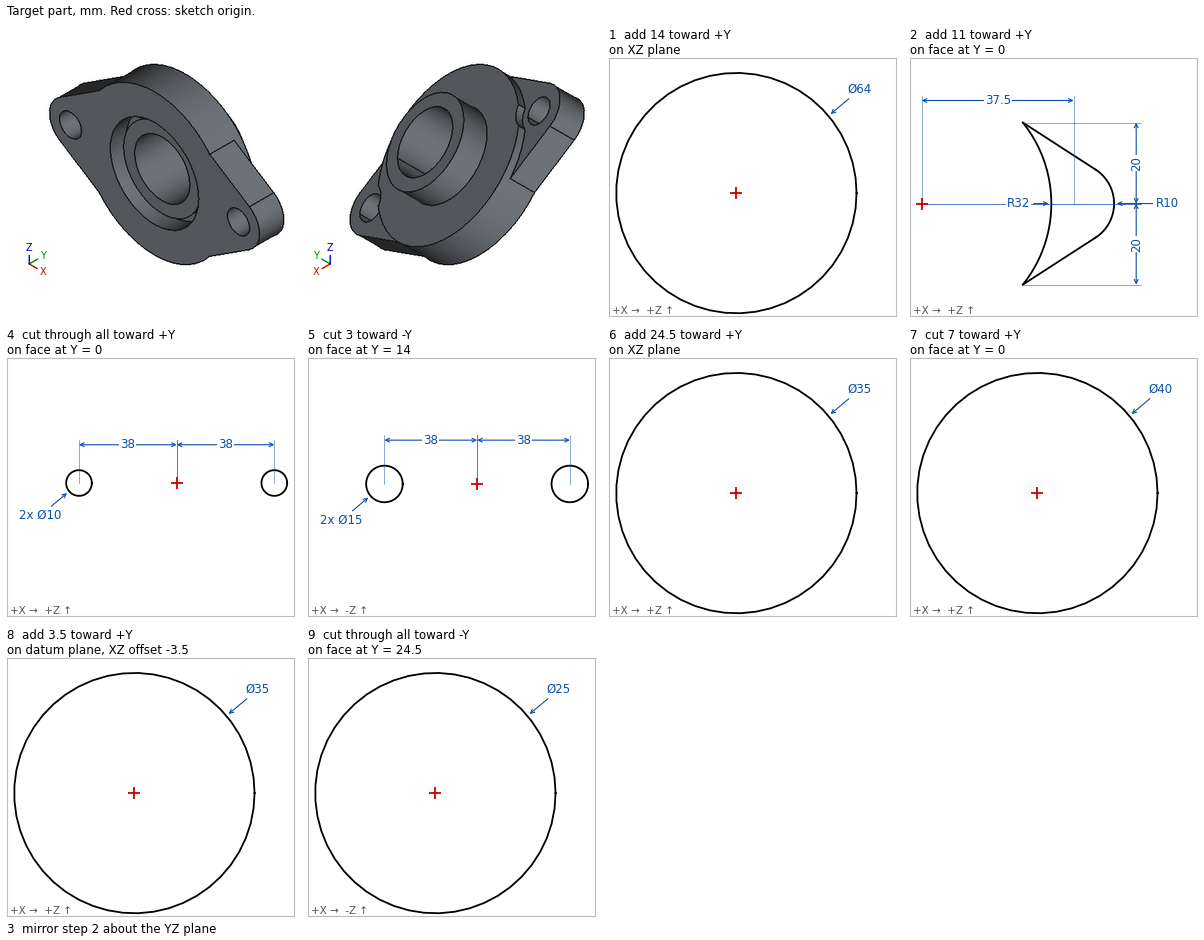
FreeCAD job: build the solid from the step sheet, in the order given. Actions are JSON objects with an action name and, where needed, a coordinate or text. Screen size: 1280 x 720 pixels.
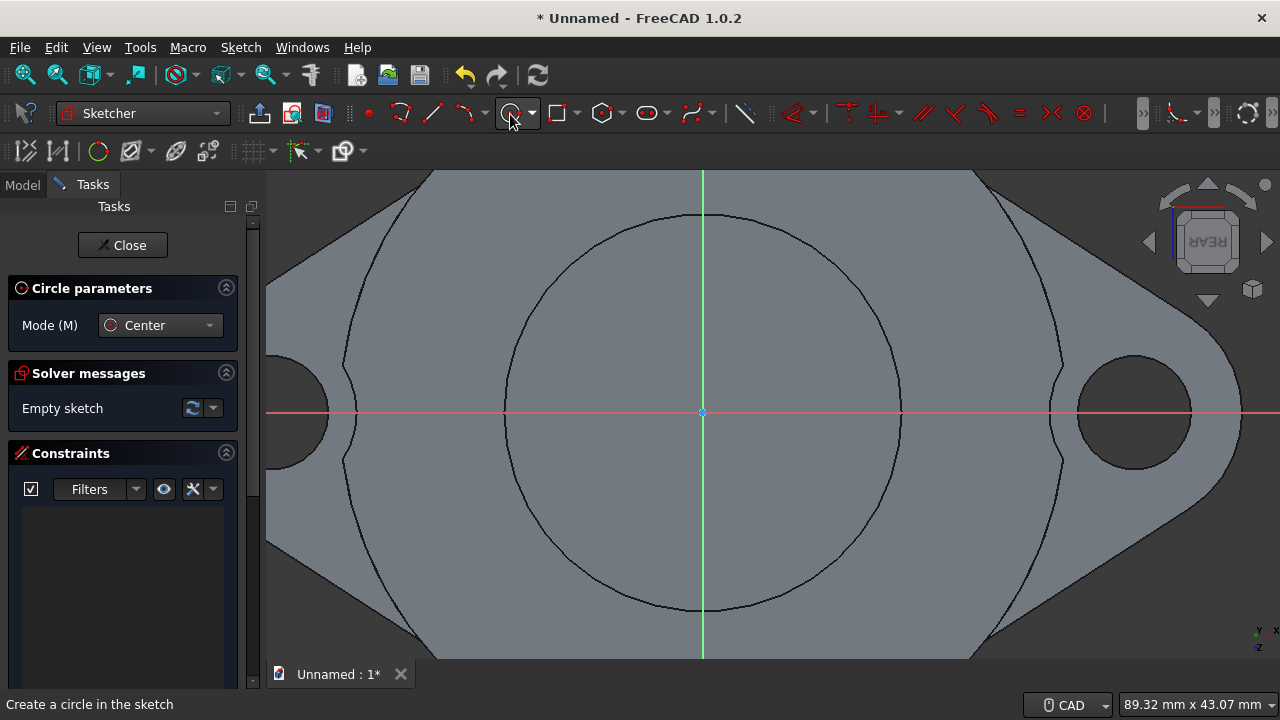
{"action": "left_click", "coordinate": [703, 413]}
{"action": "left_click", "coordinate": [803, 312]}
{"action": "key", "text": "Escape"}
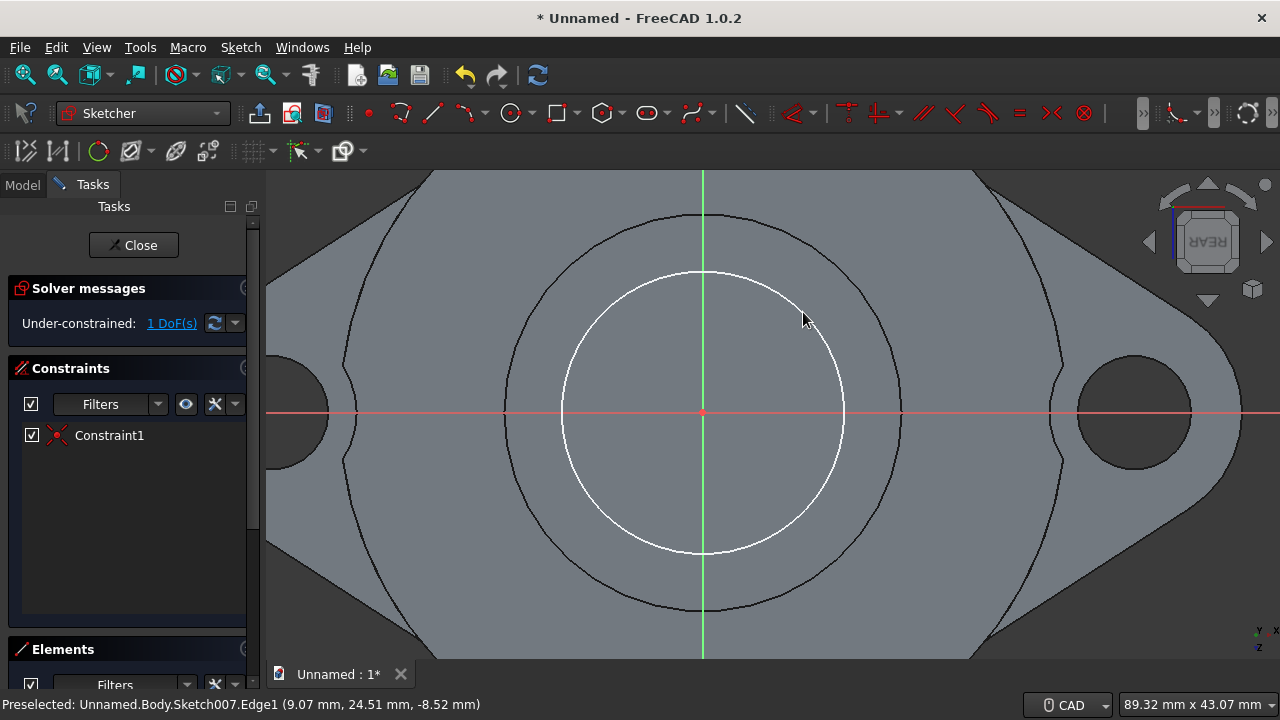
{"action": "left_click", "coordinate": [792, 114]}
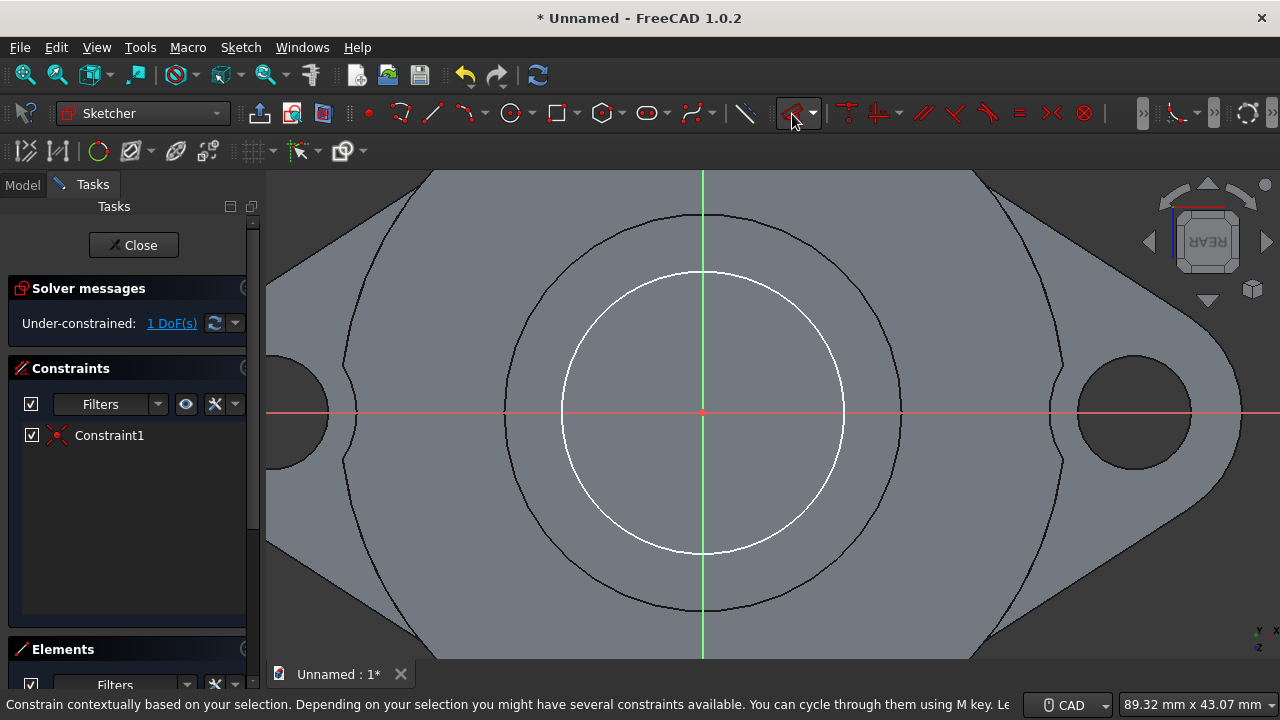
{"action": "left_click", "coordinate": [803, 313]}
{"action": "left_click", "coordinate": [826, 290]}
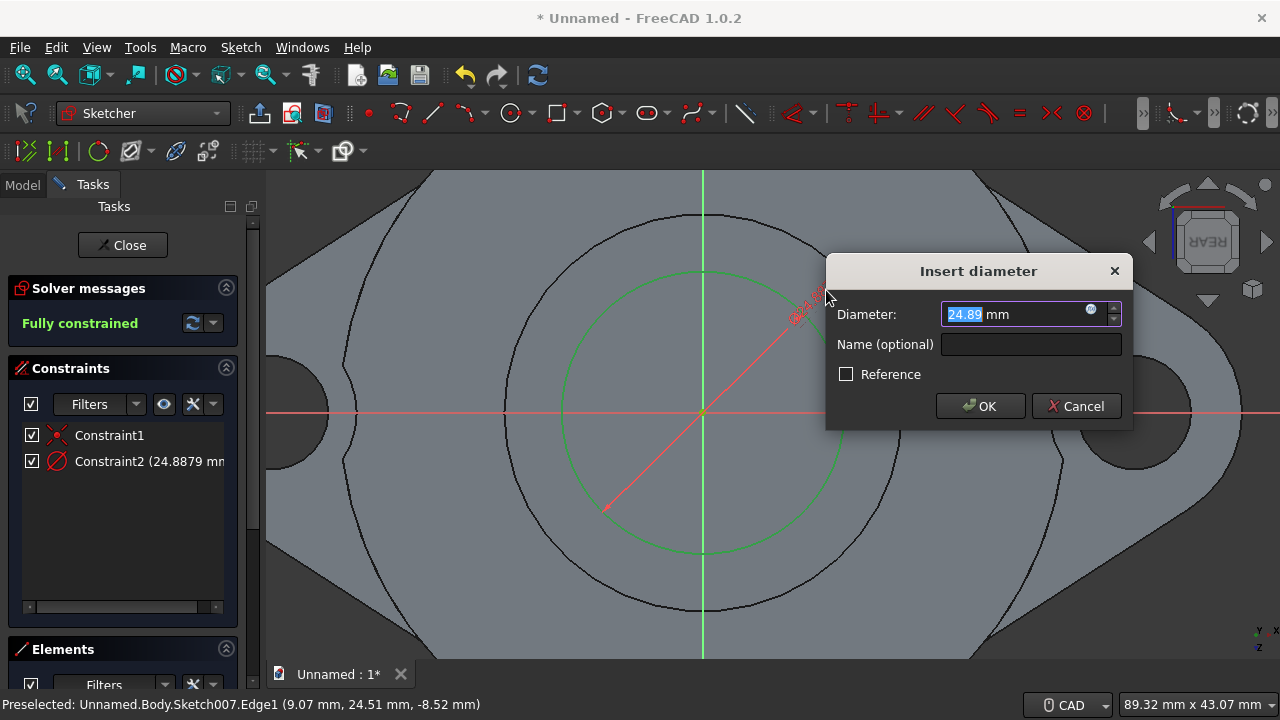
{"action": "type", "text": "25"}
{"action": "key", "text": "Return"}
{"action": "key", "text": "Escape"}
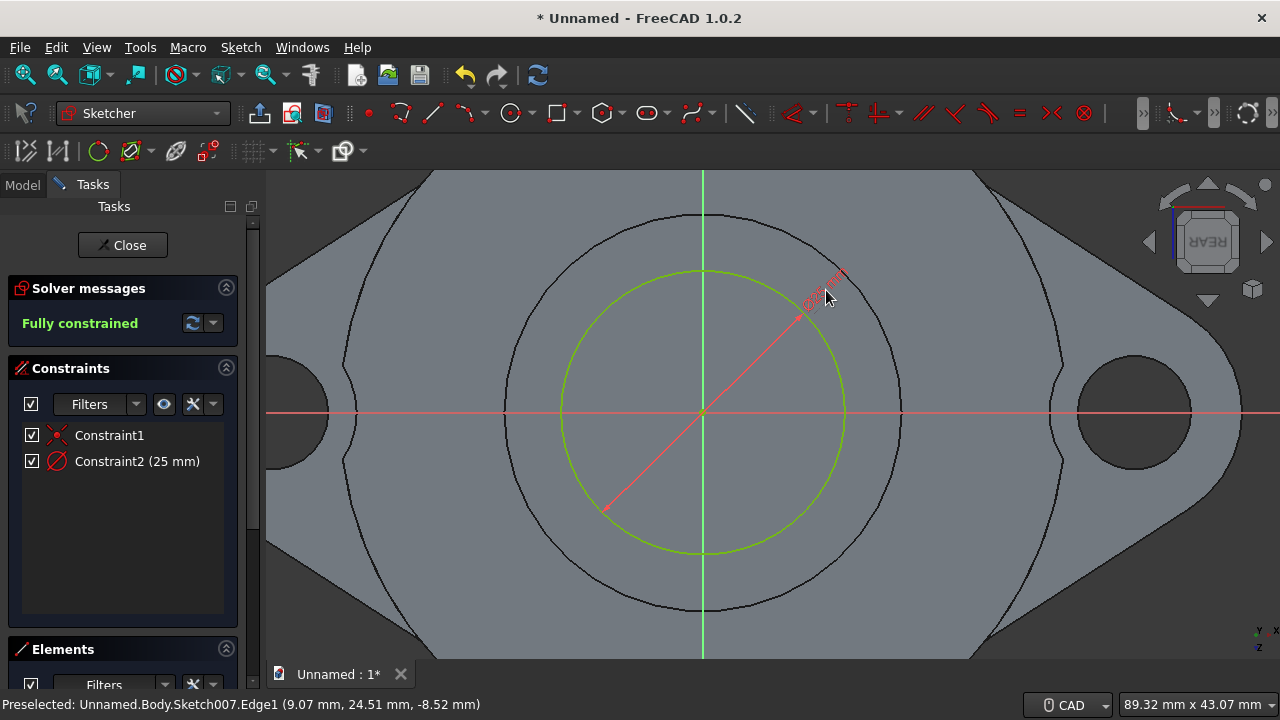
{"action": "left_click", "coordinate": [123, 245]}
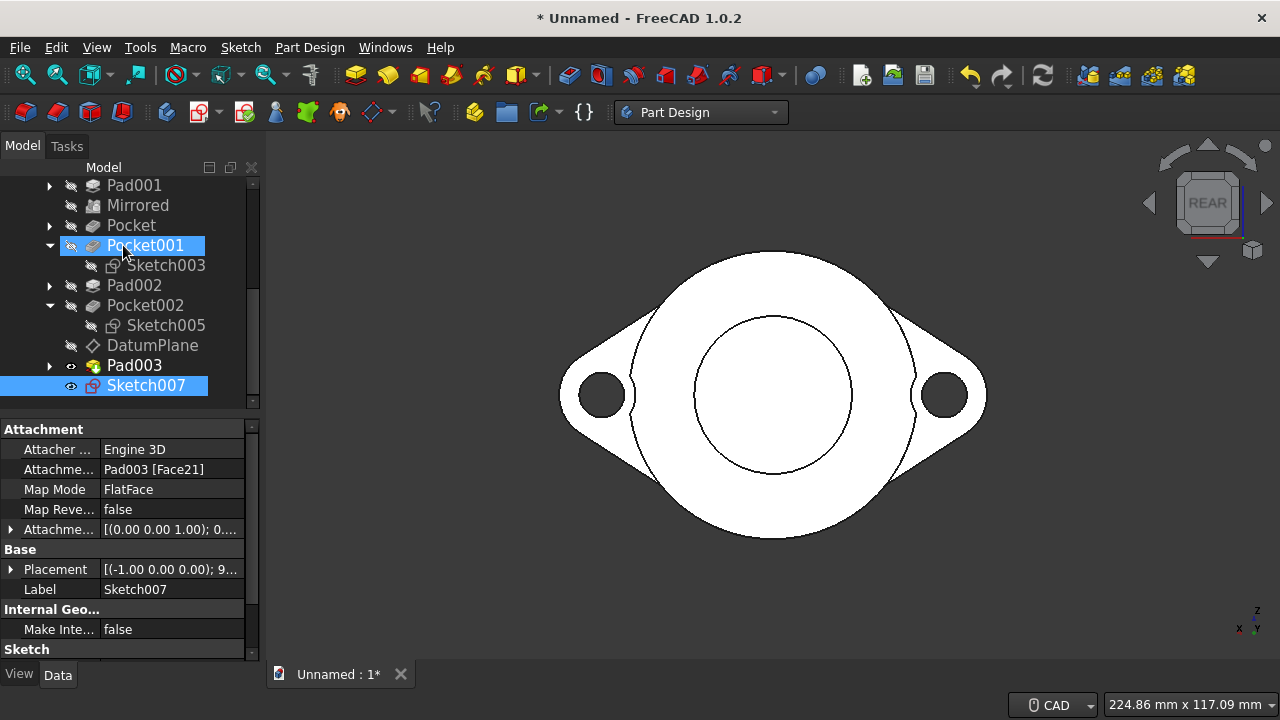
{"action": "left_click", "coordinate": [570, 76]}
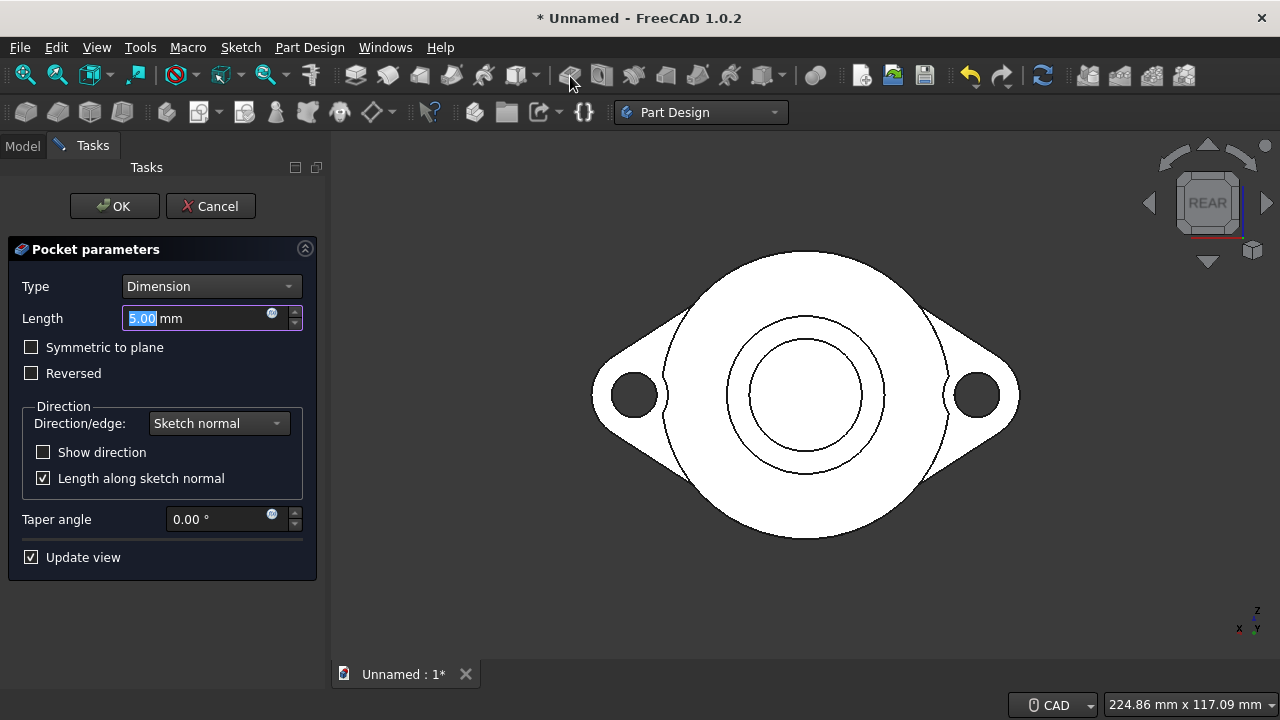
{"action": "left_click", "coordinate": [212, 286]}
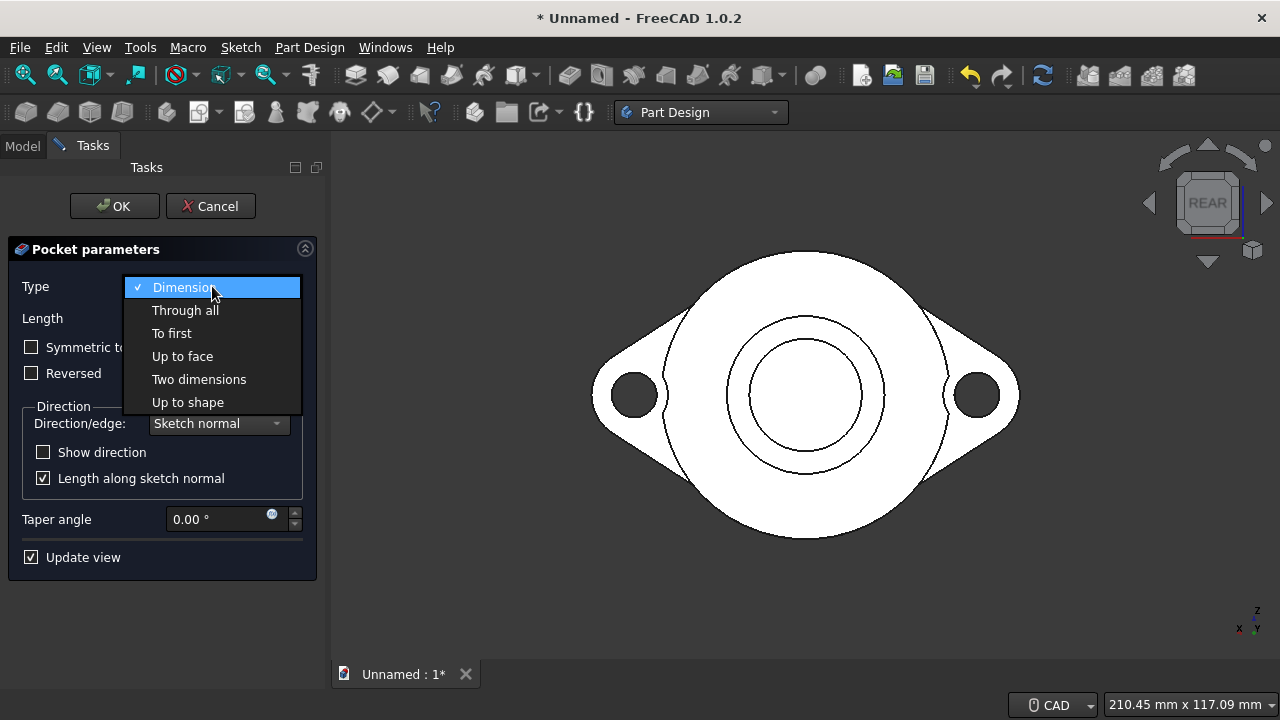
{"action": "left_click", "coordinate": [212, 310]}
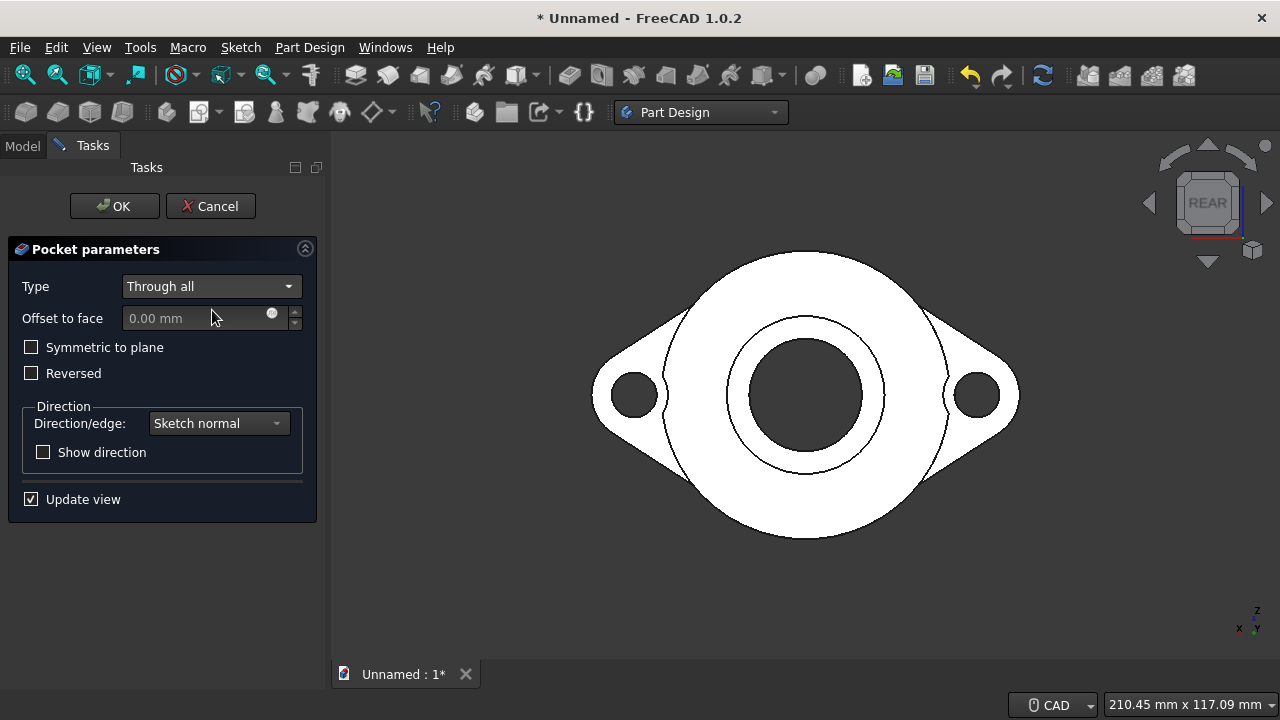
{"action": "left_click", "coordinate": [115, 206]}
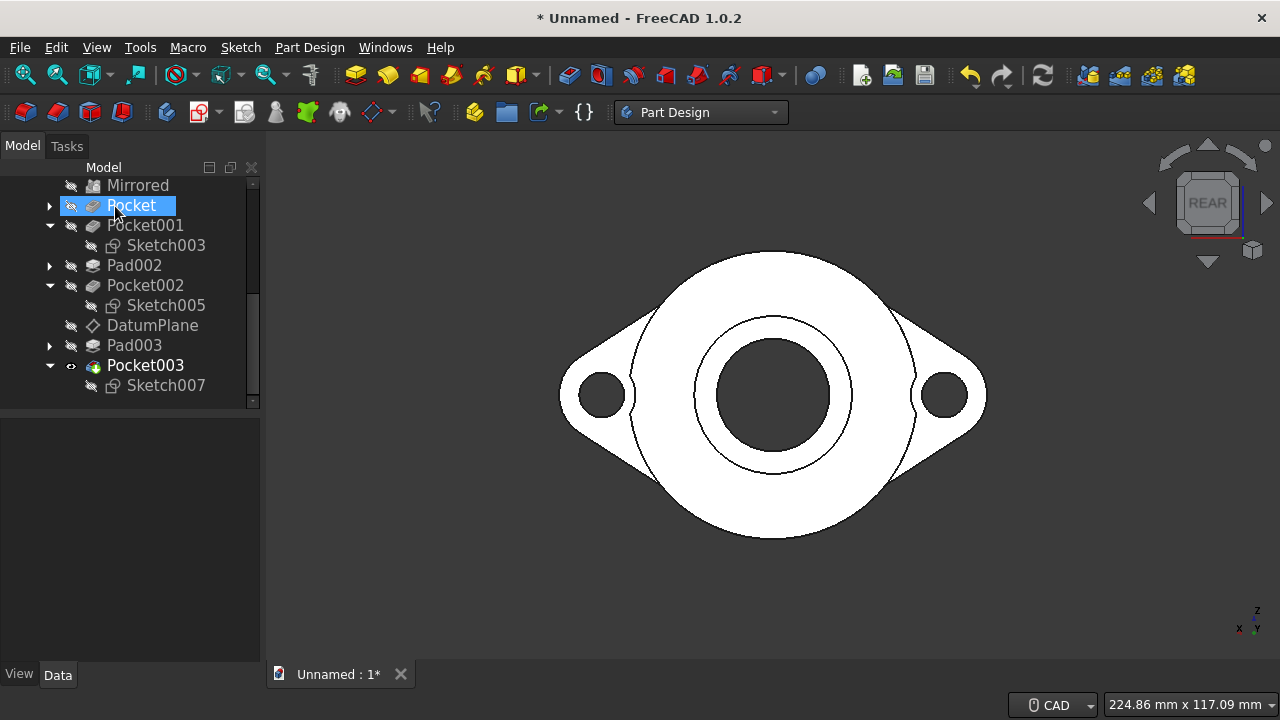
{"action": "key", "text": "0"}